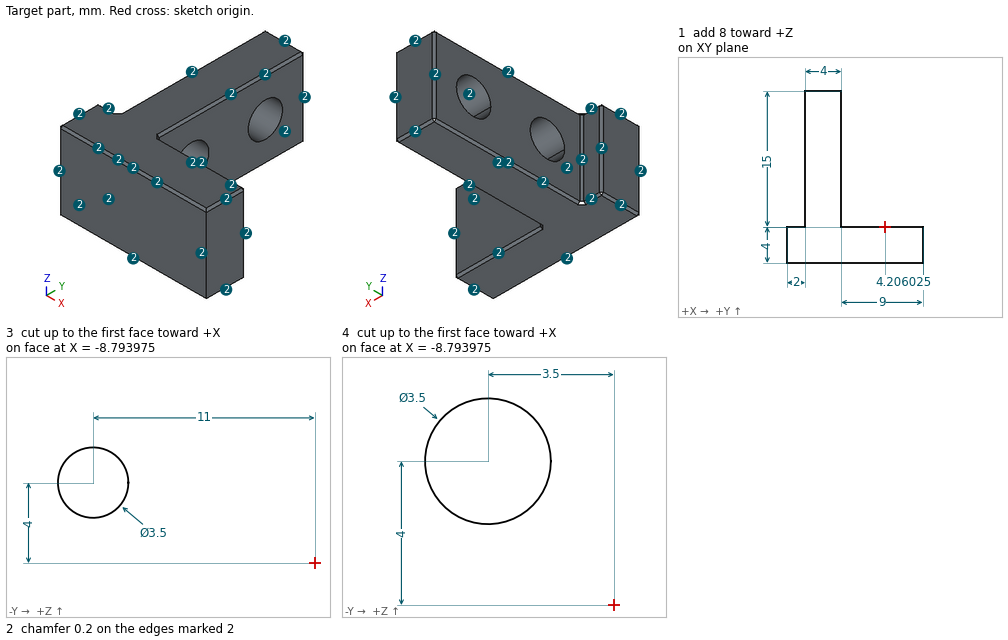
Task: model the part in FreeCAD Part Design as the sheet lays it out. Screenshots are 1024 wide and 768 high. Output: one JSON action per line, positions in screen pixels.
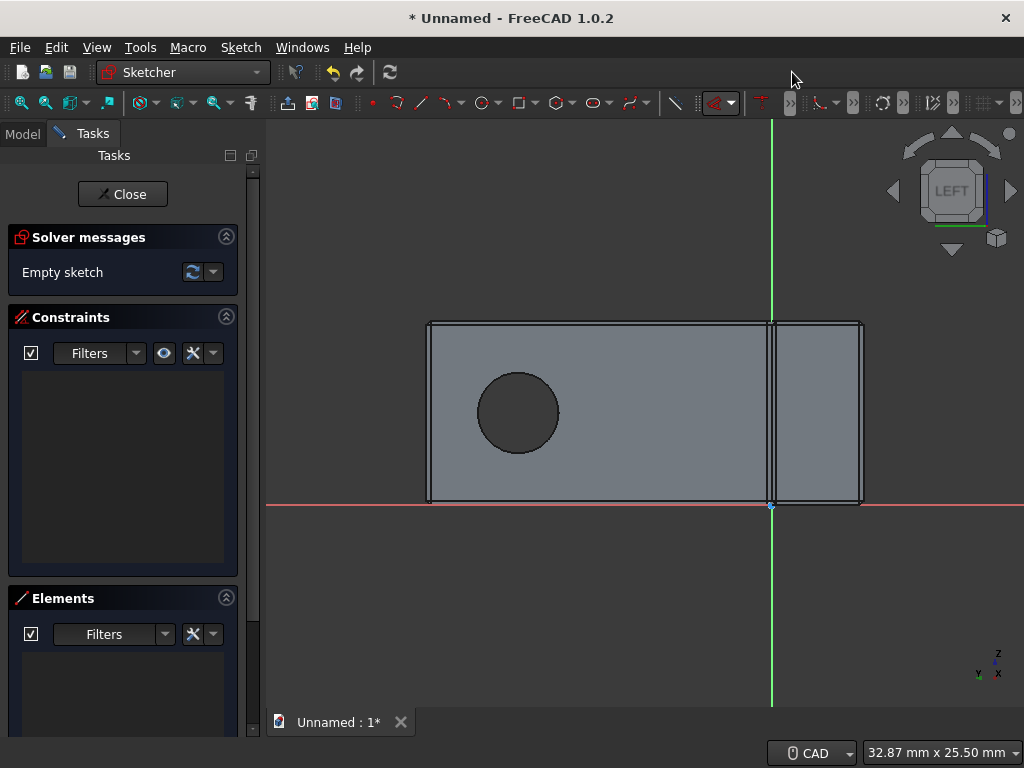
{"action": "scroll", "coordinate": [790, 454], "scroll_direction": "up", "scroll_amount": 5}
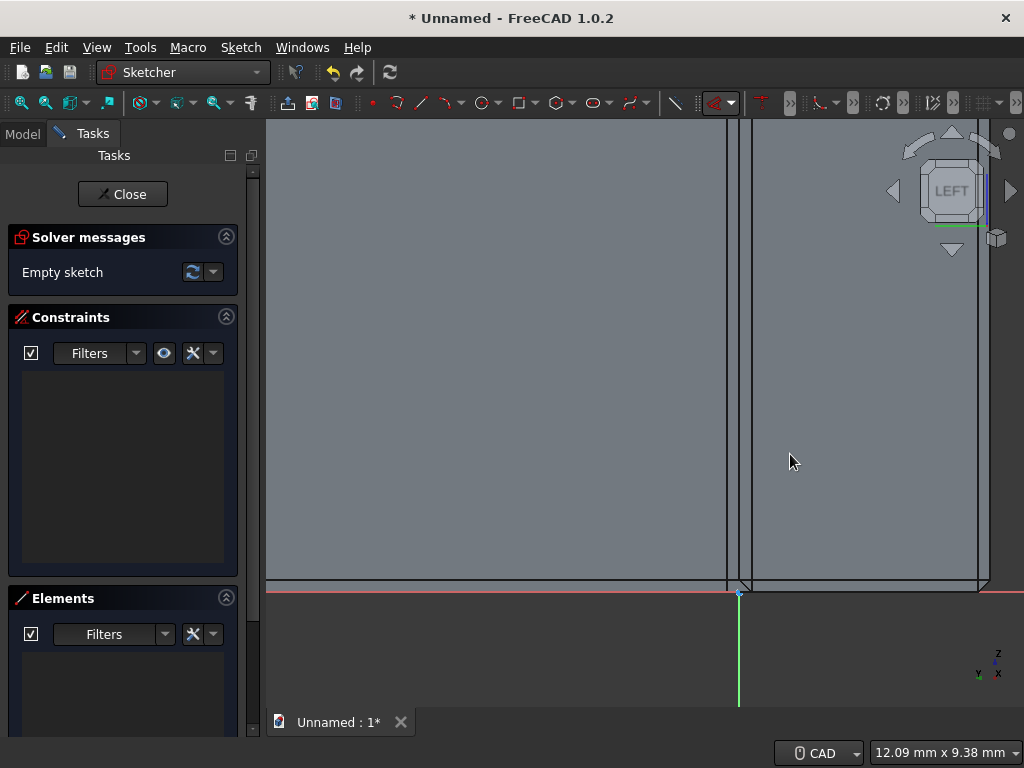
{"action": "left_click", "coordinate": [482, 104]}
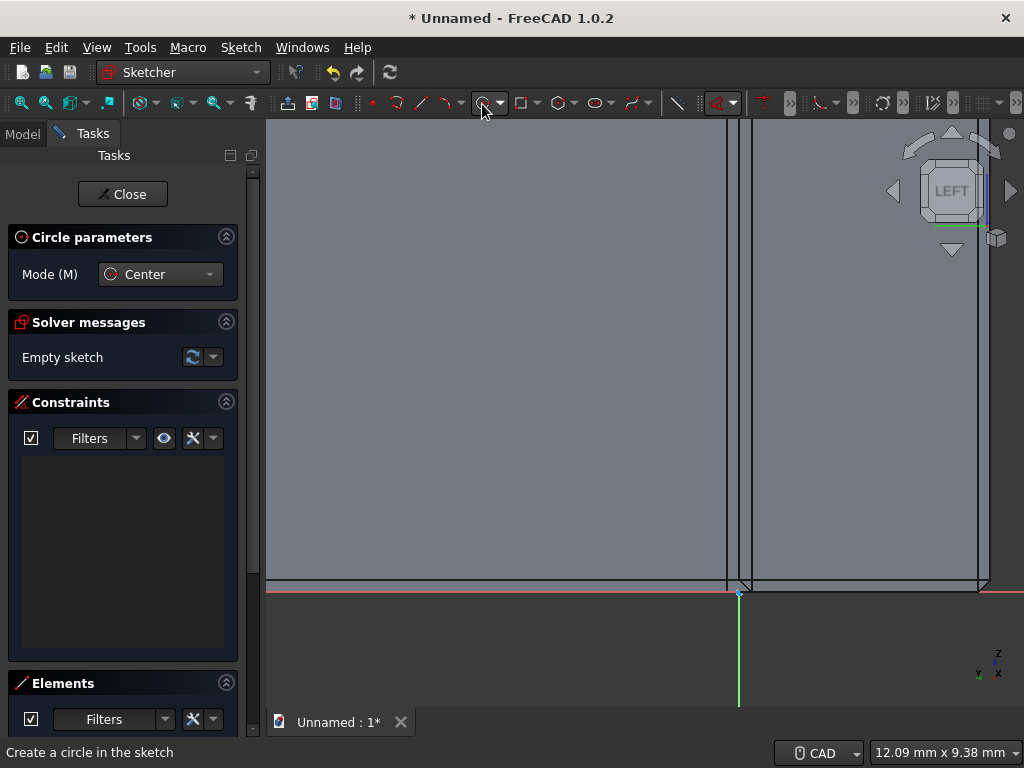
{"action": "left_click", "coordinate": [520, 342]}
{"action": "left_click", "coordinate": [598, 264]}
{"action": "key", "text": "Escape"}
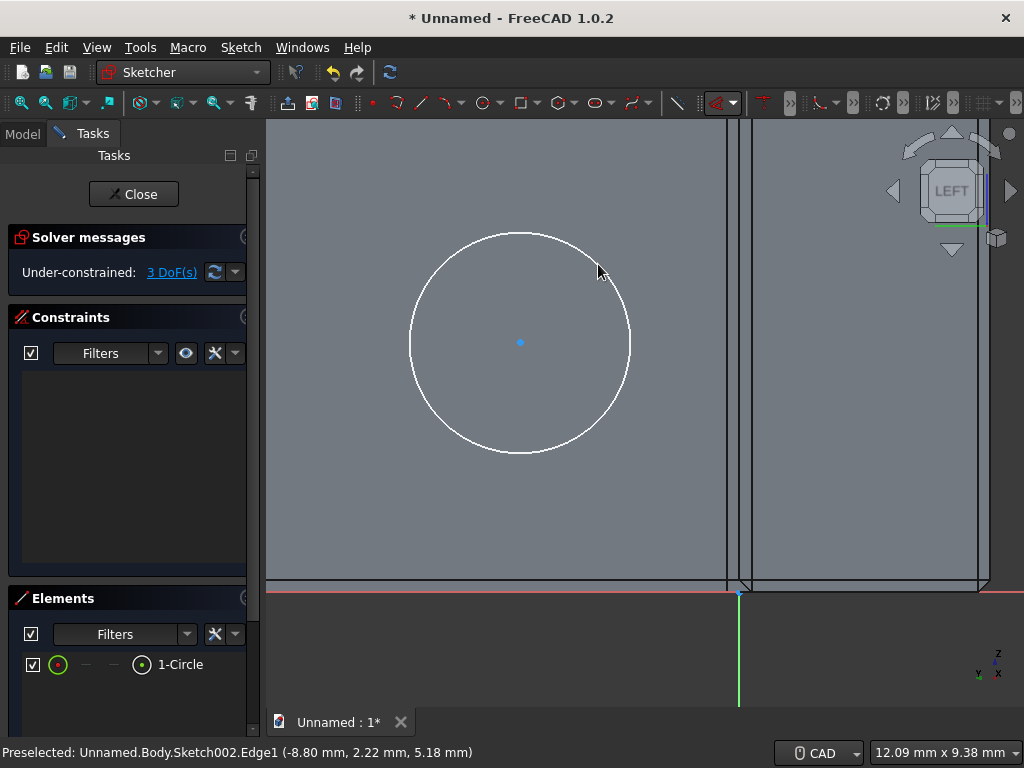
{"action": "left_click", "coordinate": [598, 265]}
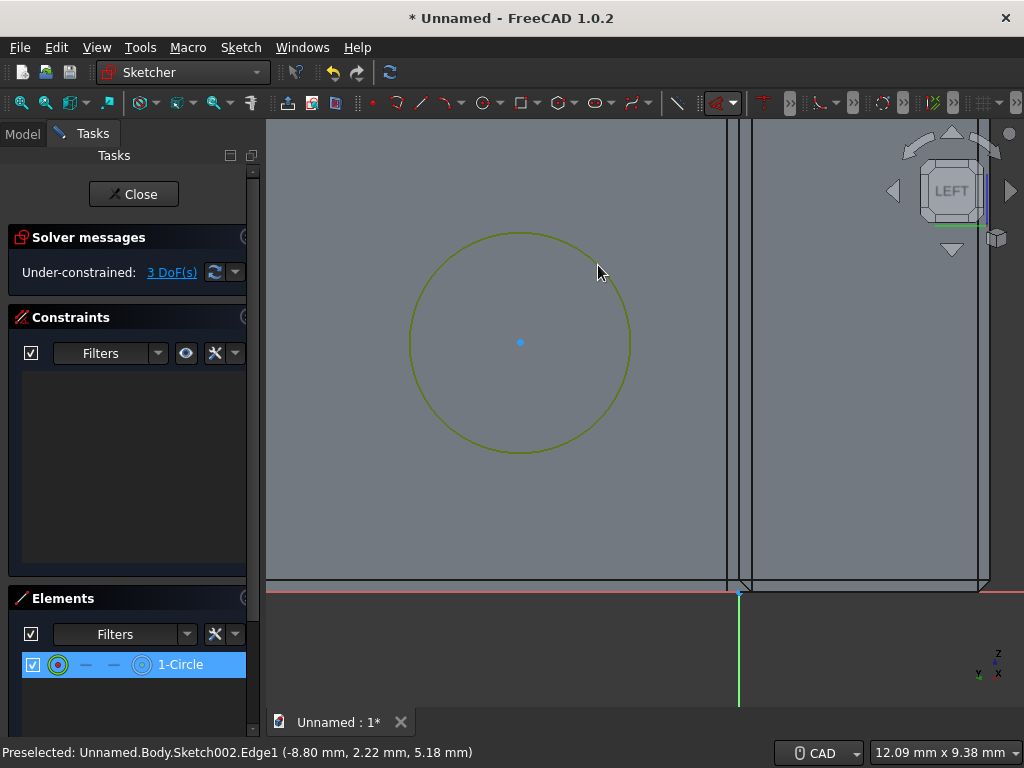
{"action": "key", "text": "k o"}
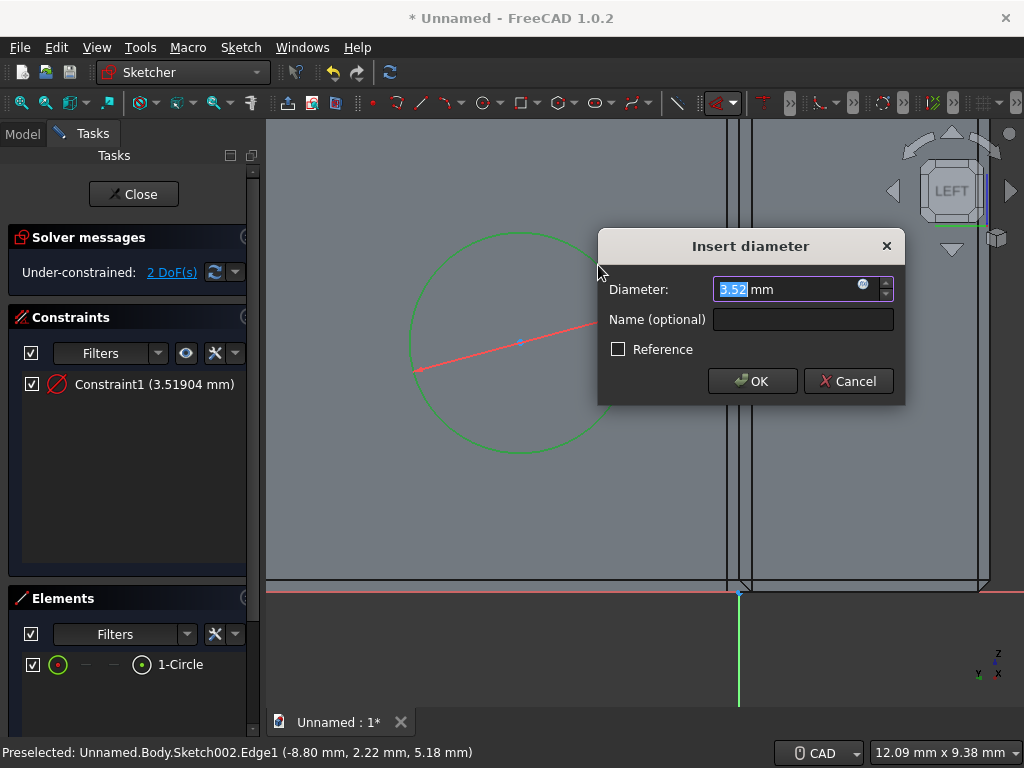
{"action": "type", "text": "3.5"}
{"action": "key", "text": "Return"}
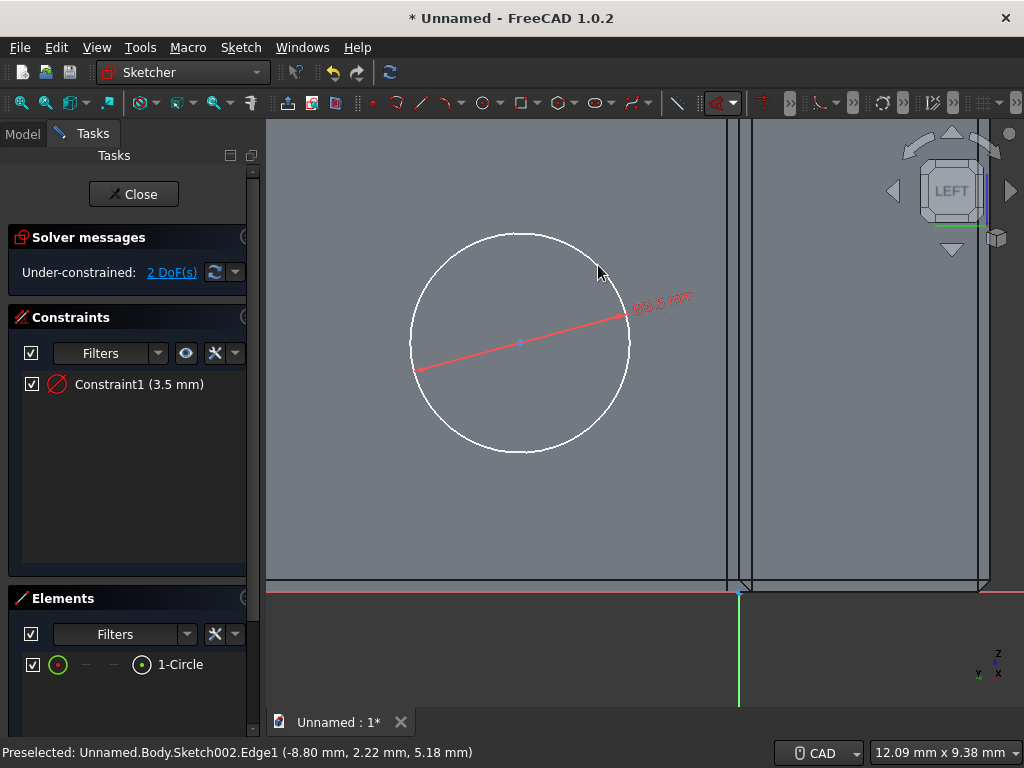
{"action": "left_click", "coordinate": [520, 343]}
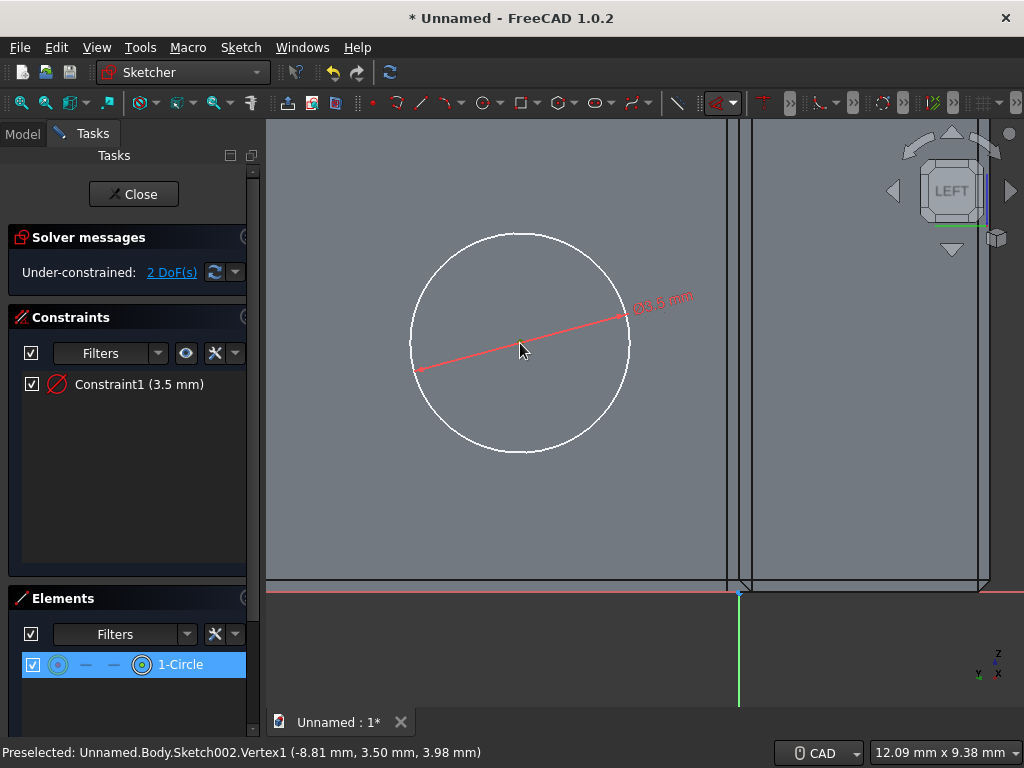
{"action": "key", "text": "i"}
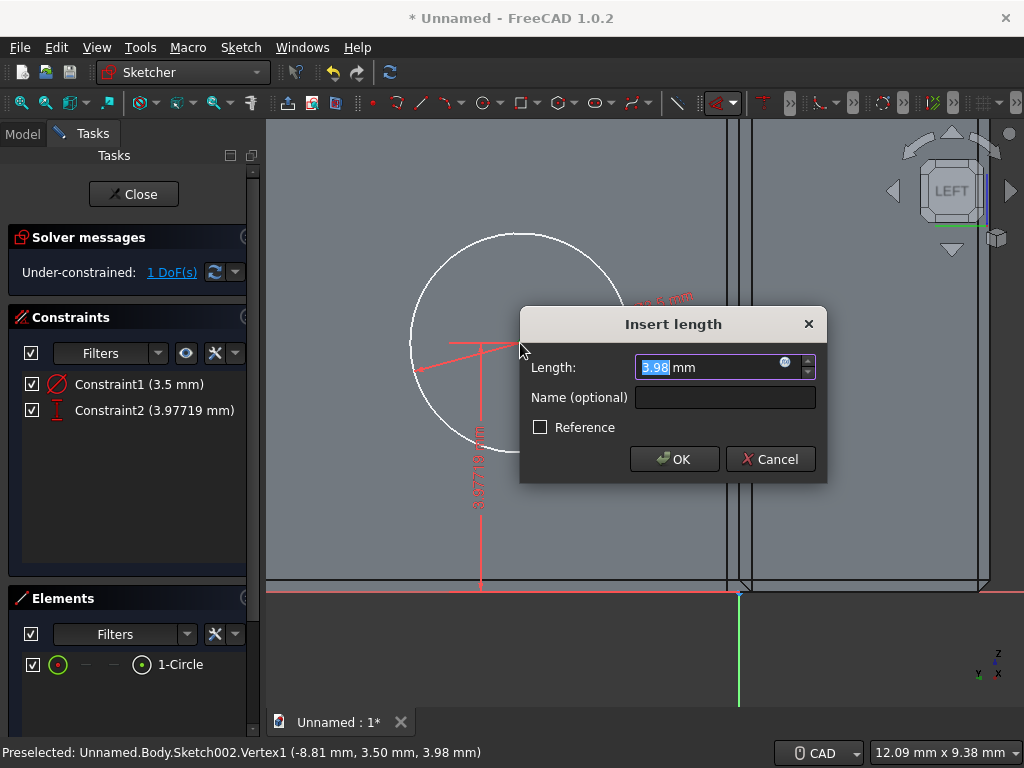
{"action": "type", "text": "4"}
{"action": "key", "text": "Return"}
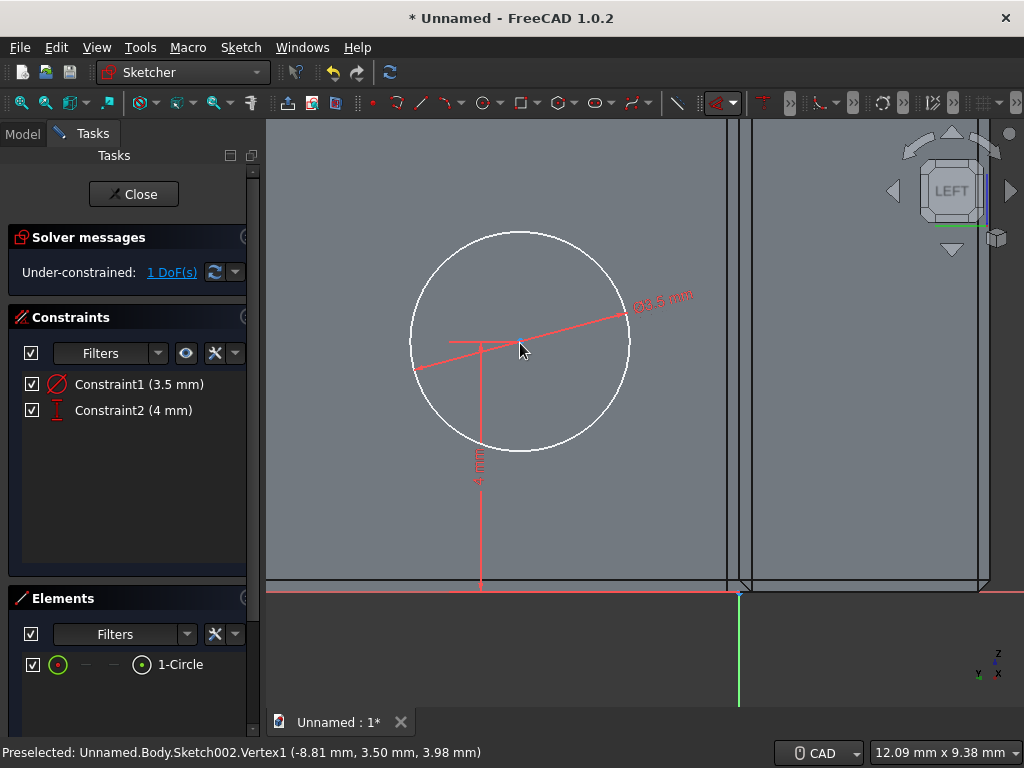
{"action": "left_click", "coordinate": [520, 342]}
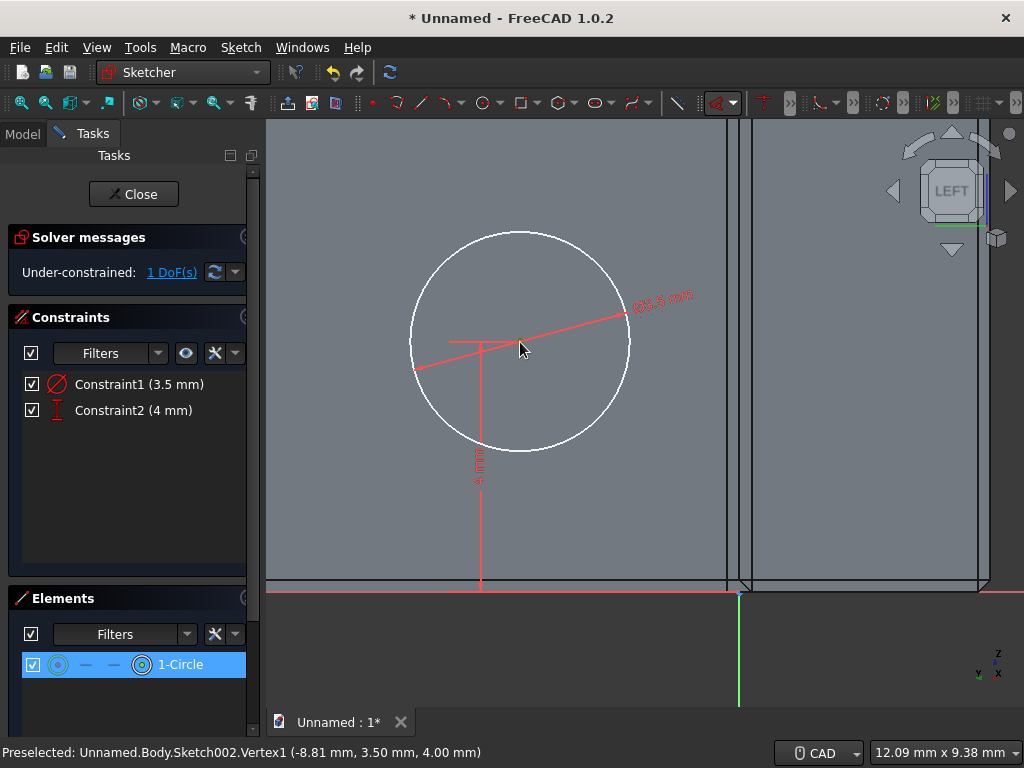
{"action": "left_click", "coordinate": [736, 104]}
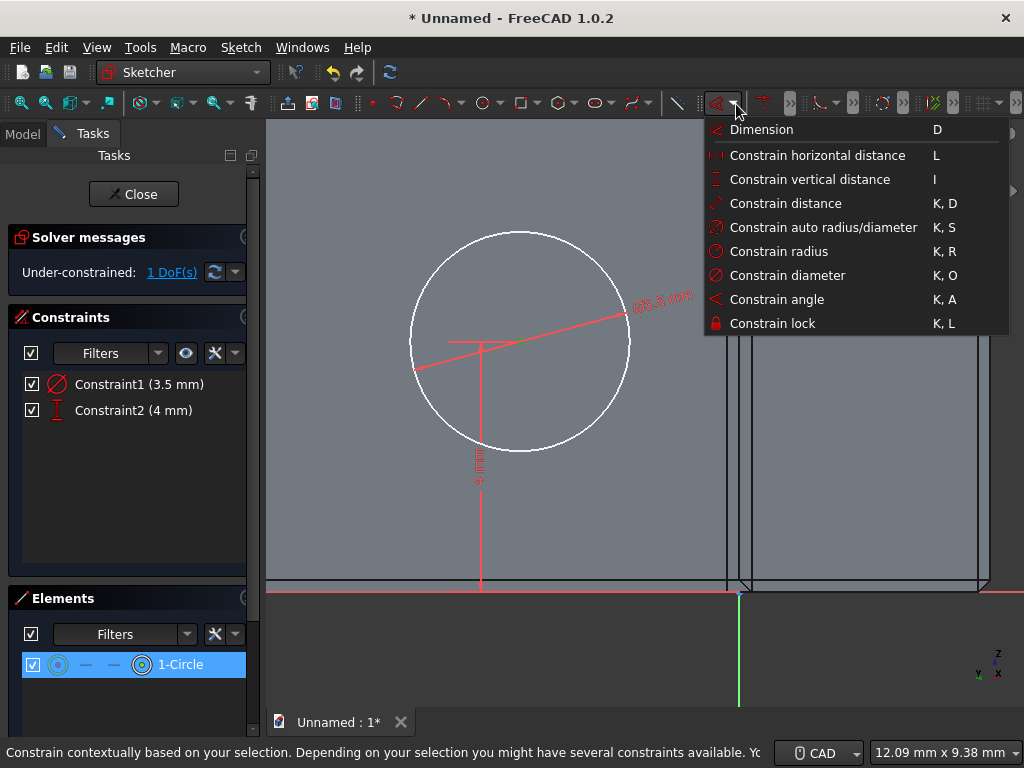
{"action": "left_click", "coordinate": [857, 155]}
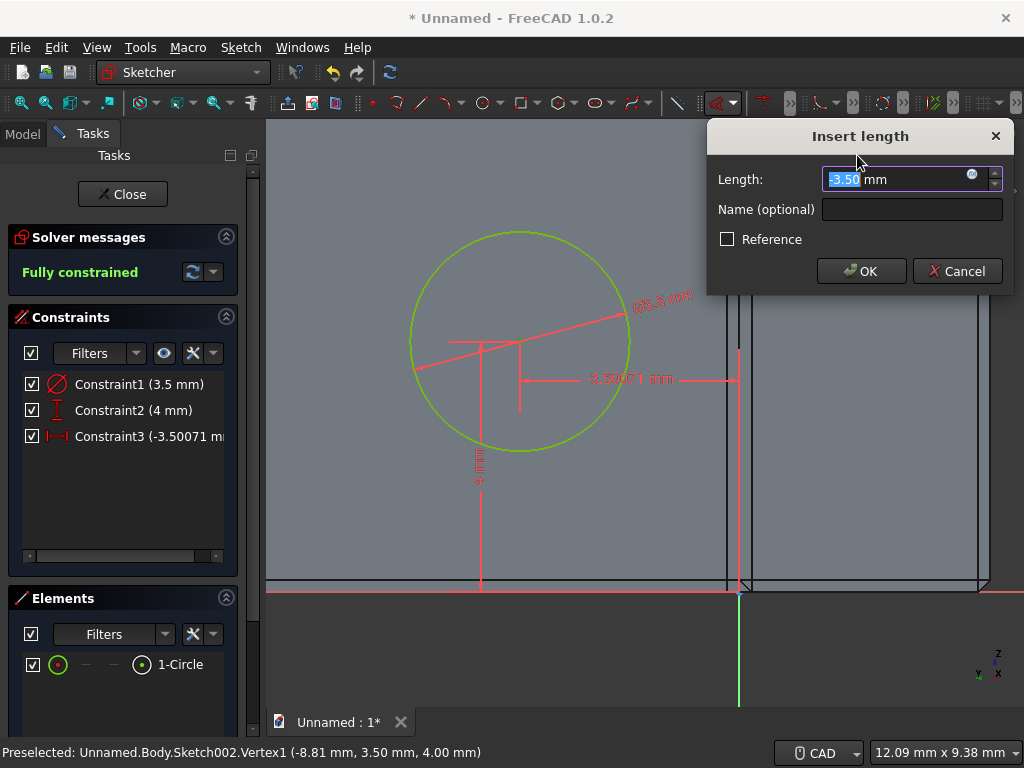
{"action": "type", "text": "-3.5"}
{"action": "key", "text": "Return"}